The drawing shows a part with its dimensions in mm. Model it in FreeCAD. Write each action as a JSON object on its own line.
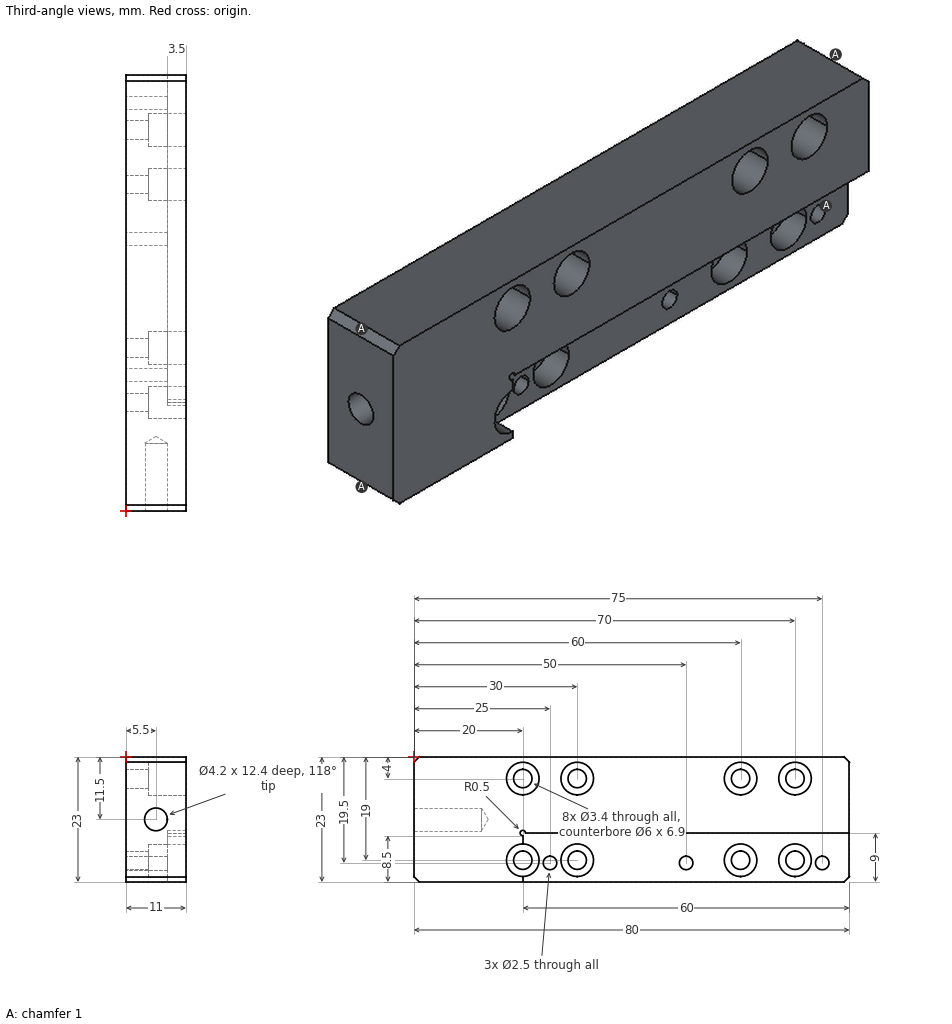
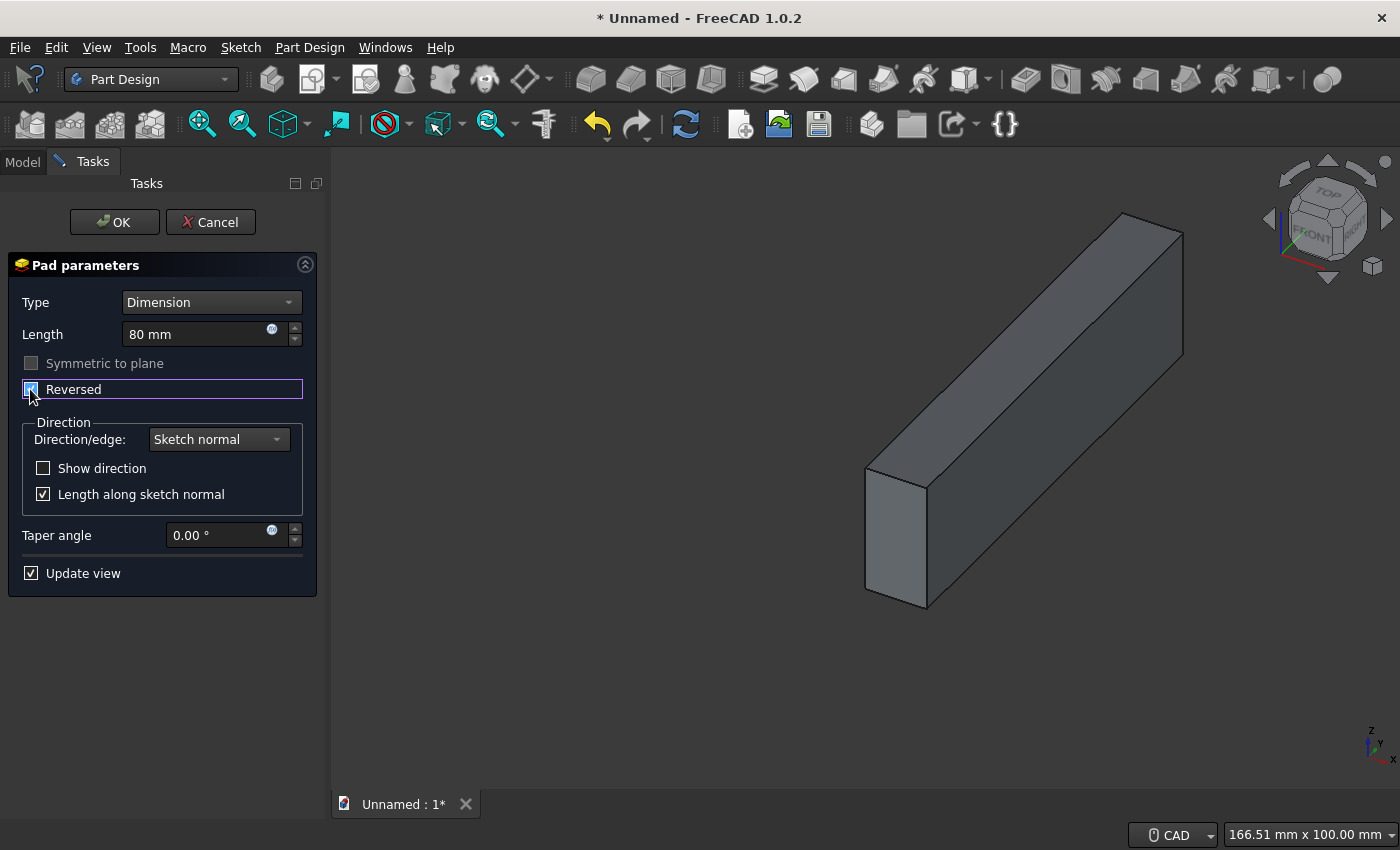
{"action": "left_click", "coordinate": [115, 222]}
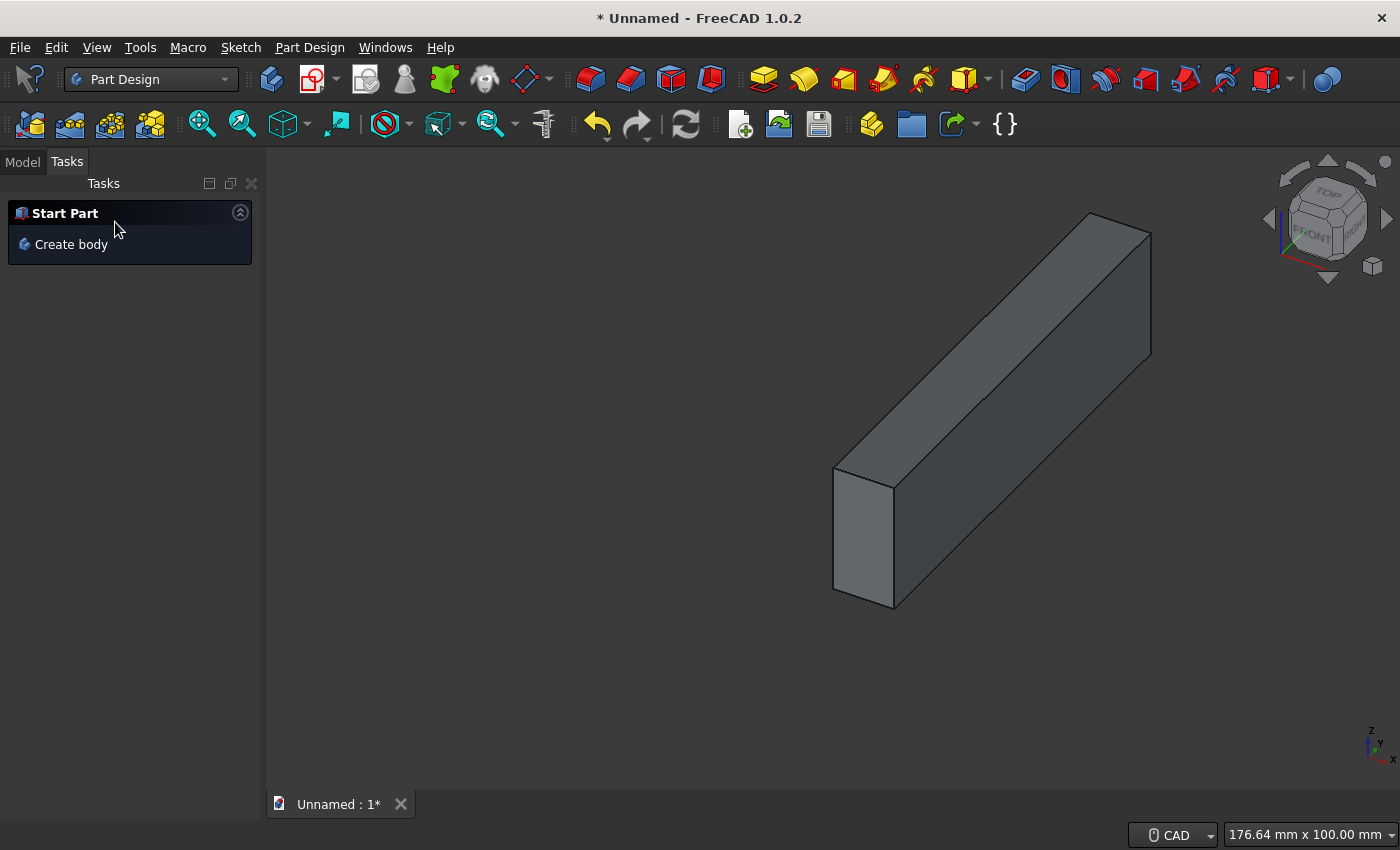
{"action": "left_click", "coordinate": [1096, 347]}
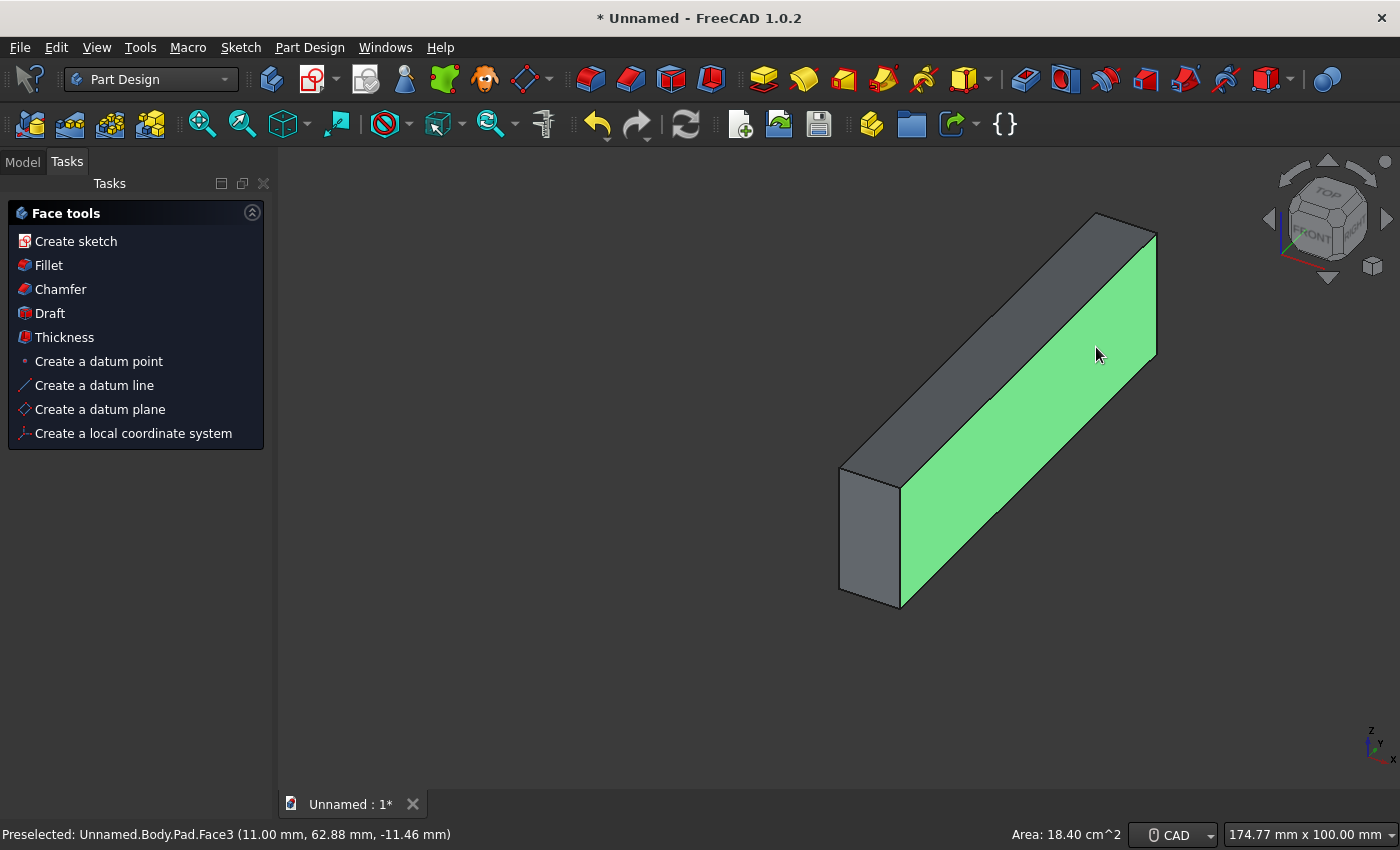
{"action": "left_click", "coordinate": [312, 80]}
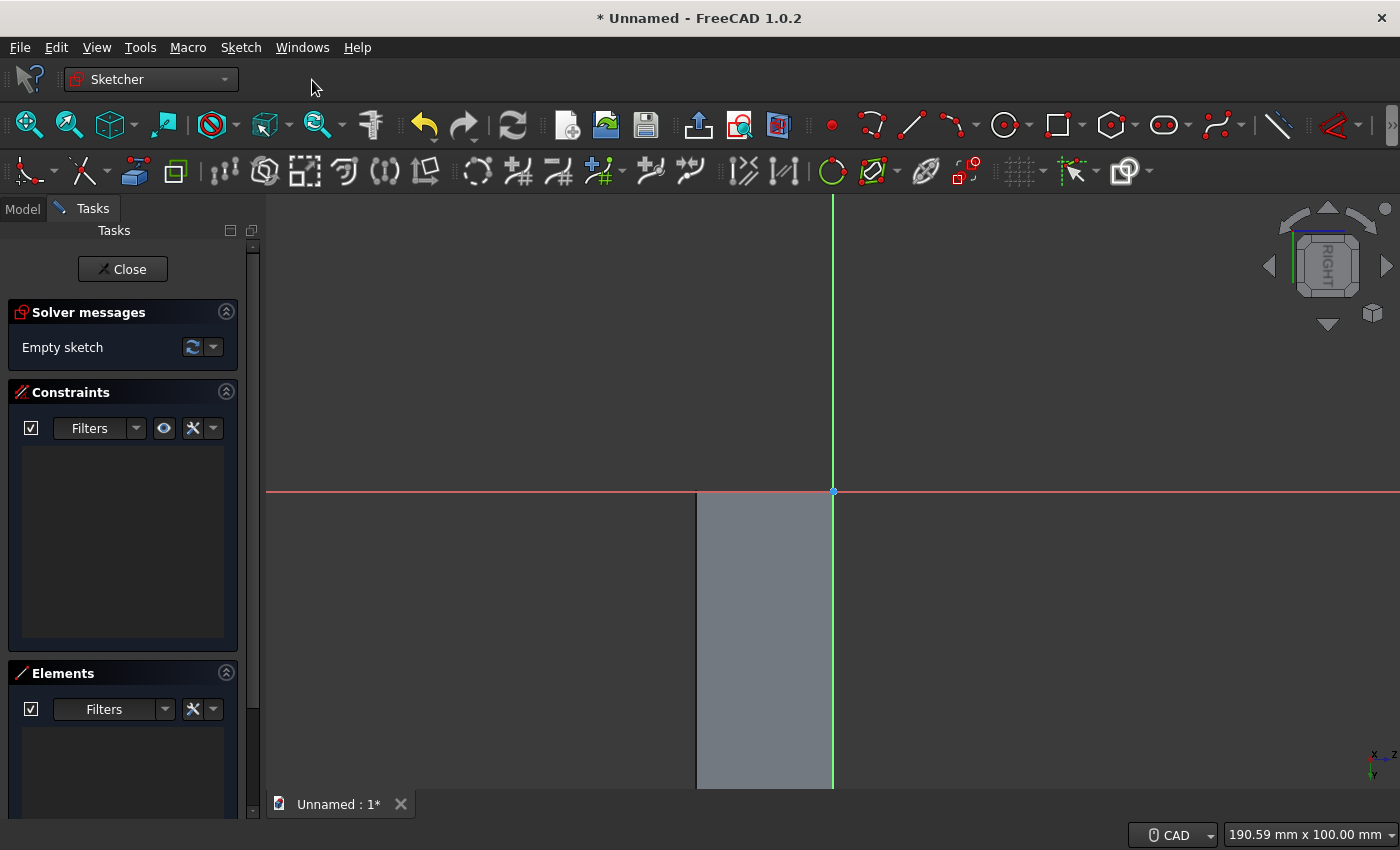
{"action": "scroll", "coordinate": [764, 222], "scroll_direction": "down", "scroll_amount": 2}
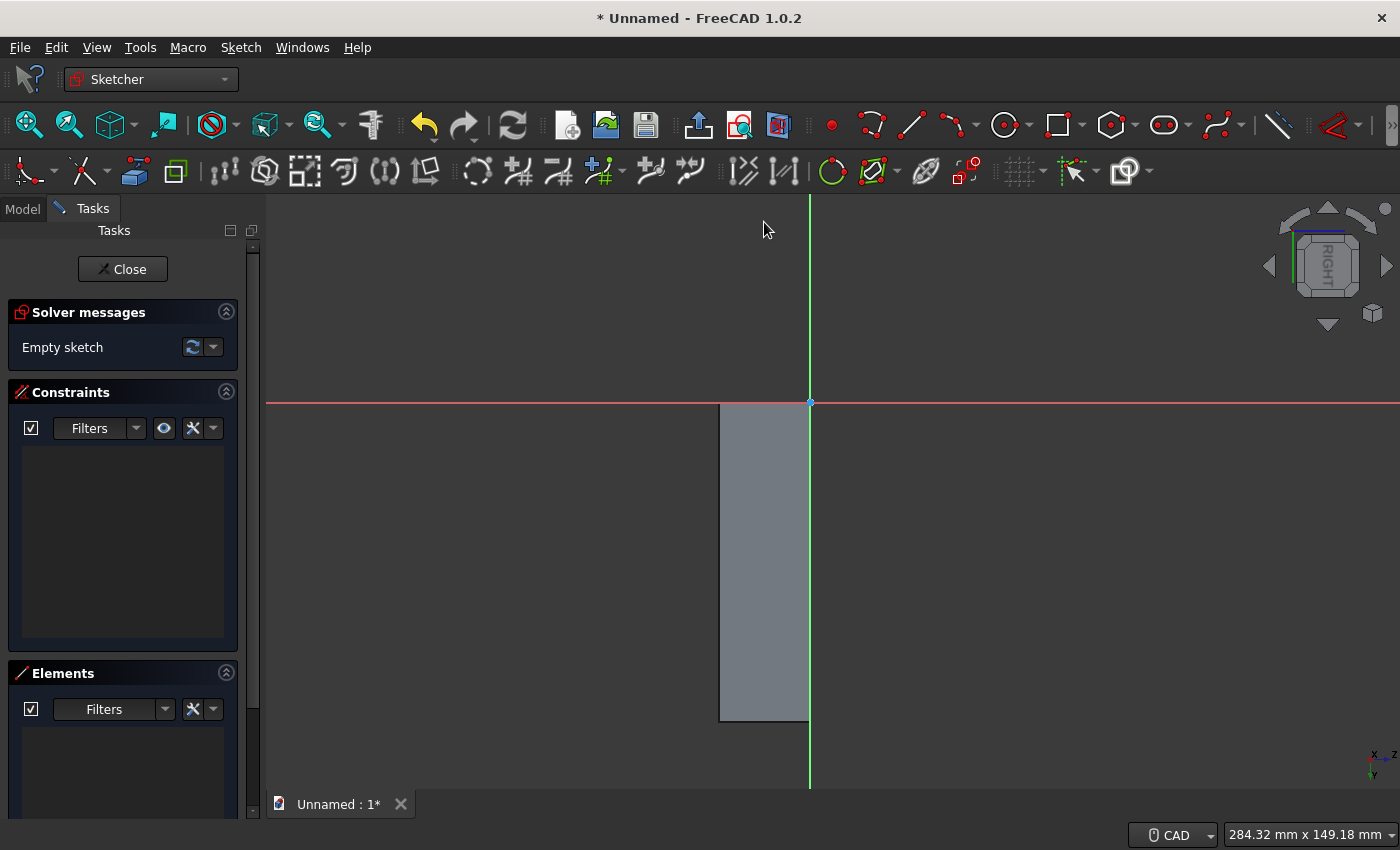
{"action": "left_click", "coordinate": [872, 126]}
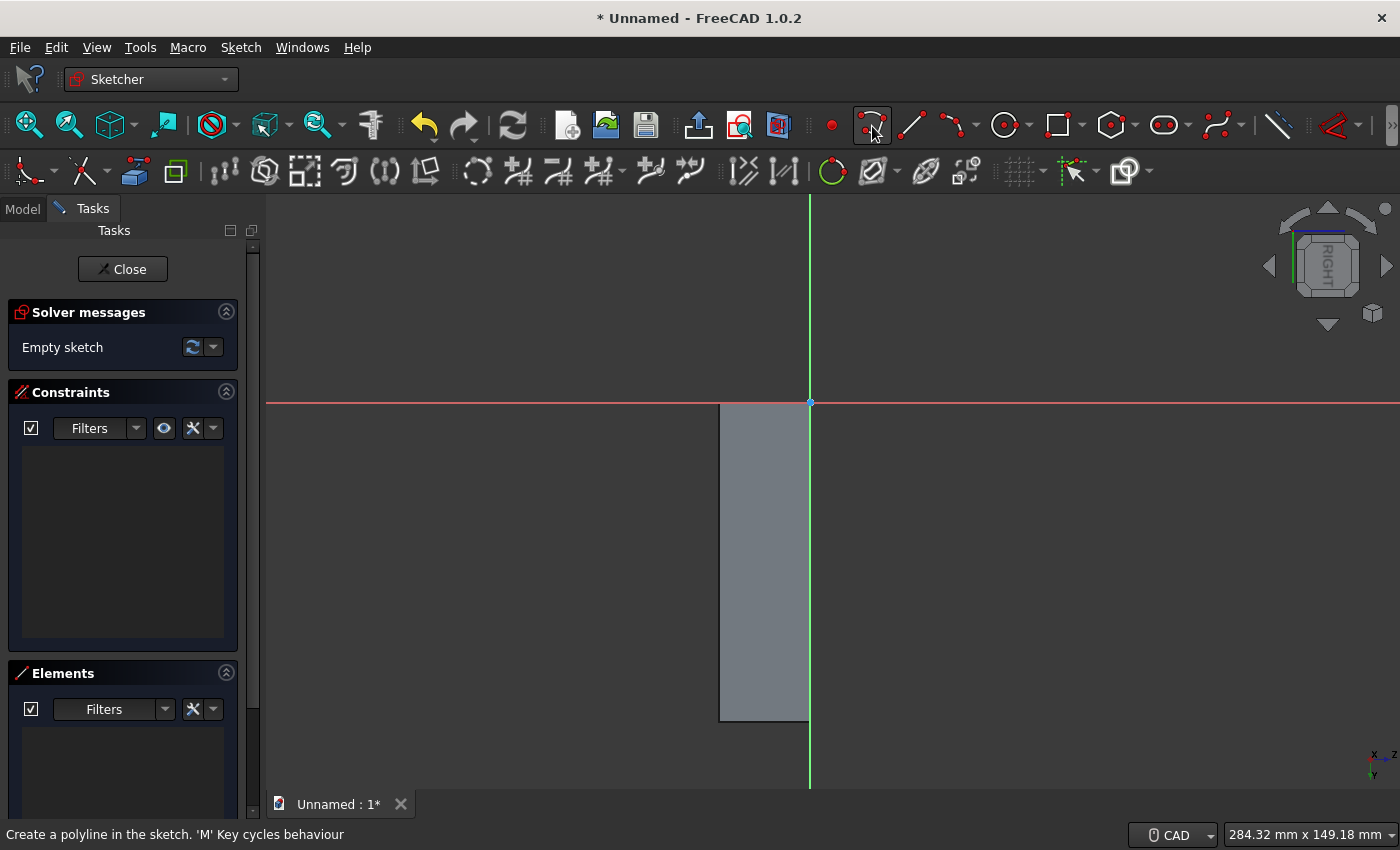
{"action": "left_click", "coordinate": [753, 482]}
{"action": "left_click", "coordinate": [719, 482]}
{"action": "left_click", "coordinate": [719, 722]}
{"action": "left_click", "coordinate": [755, 722]}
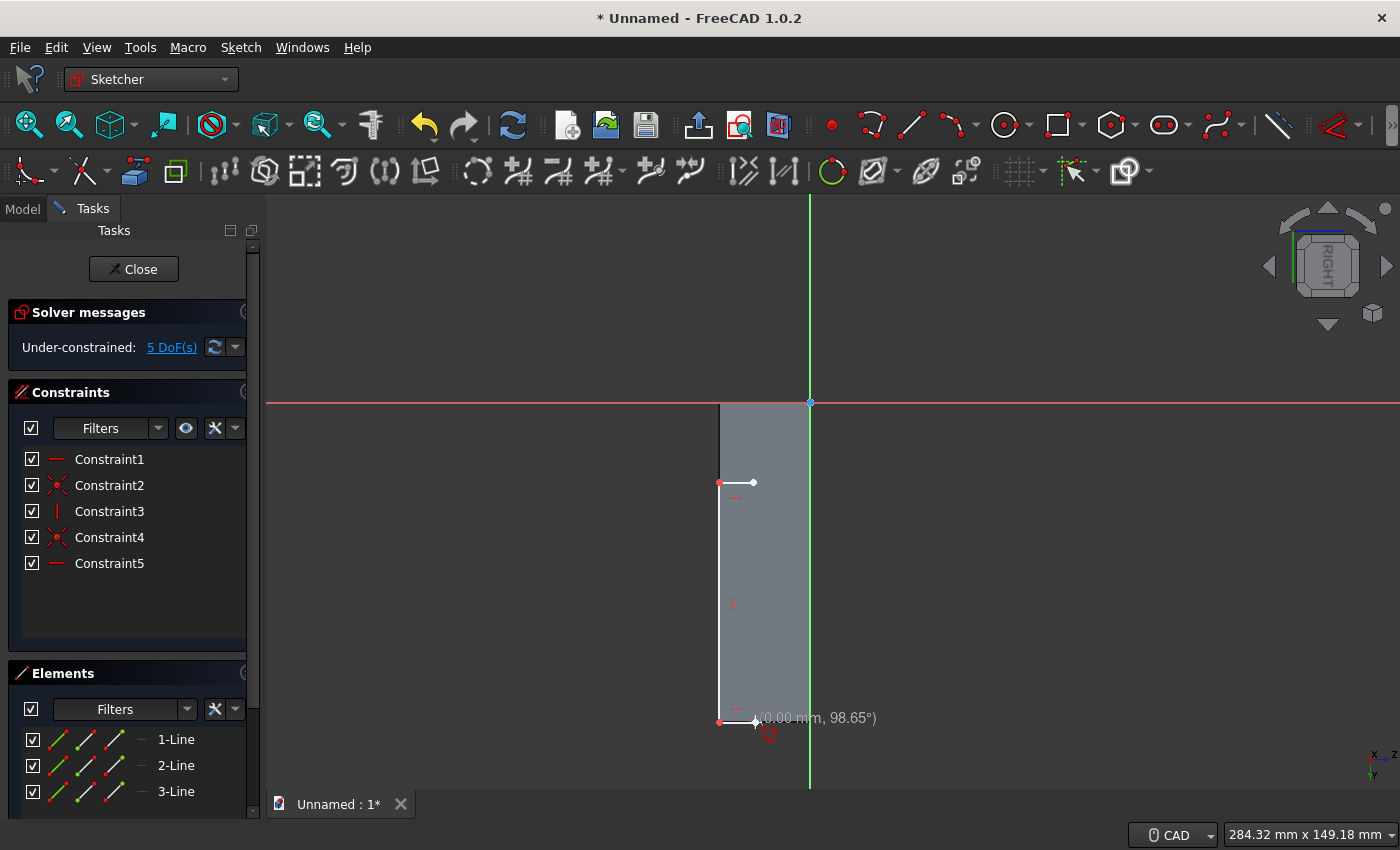
{"action": "scroll", "coordinate": [755, 484], "scroll_direction": "up", "scroll_amount": 9}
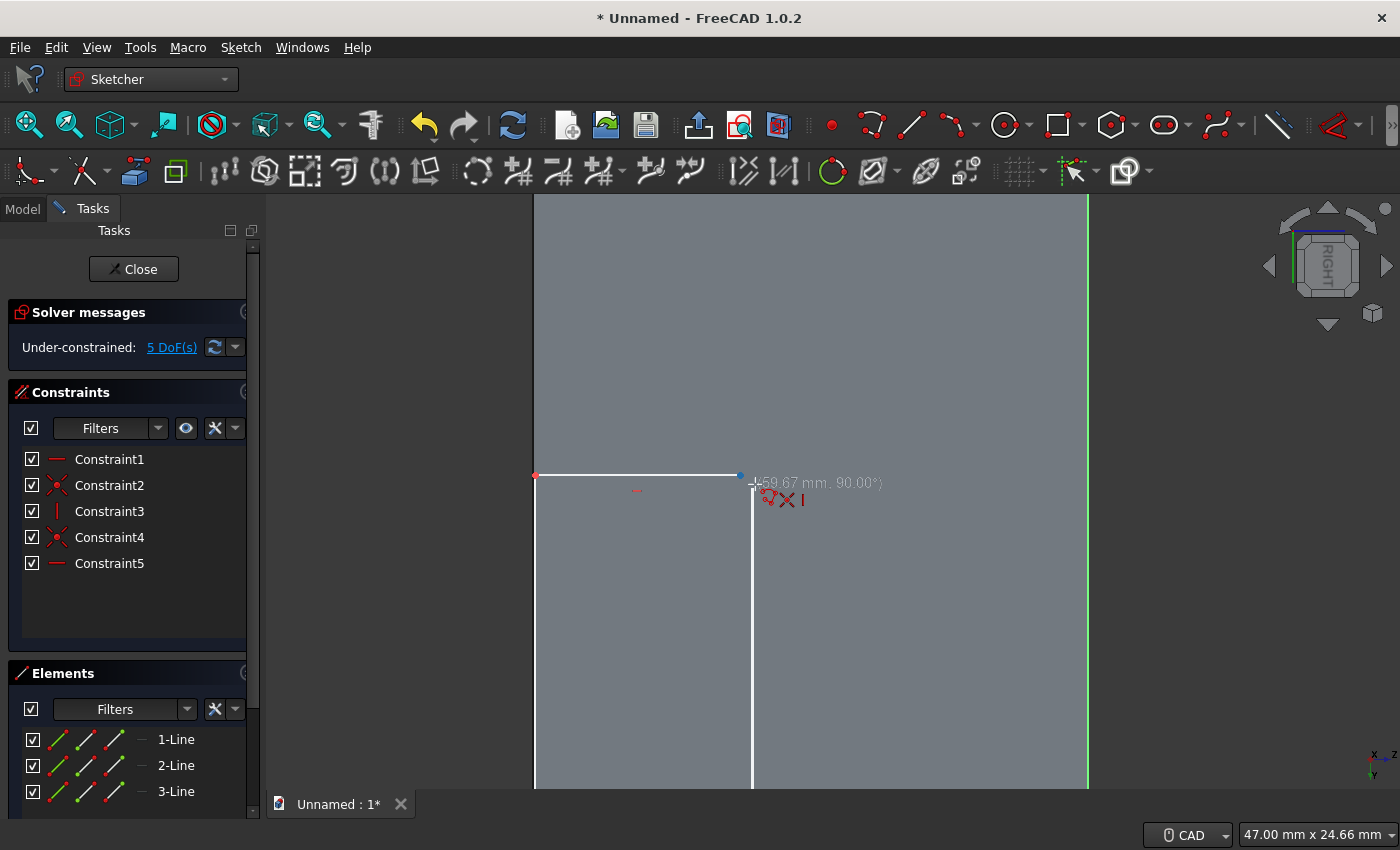
{"action": "left_click", "coordinate": [753, 484]}
{"action": "right_click", "coordinate": [753, 484]}